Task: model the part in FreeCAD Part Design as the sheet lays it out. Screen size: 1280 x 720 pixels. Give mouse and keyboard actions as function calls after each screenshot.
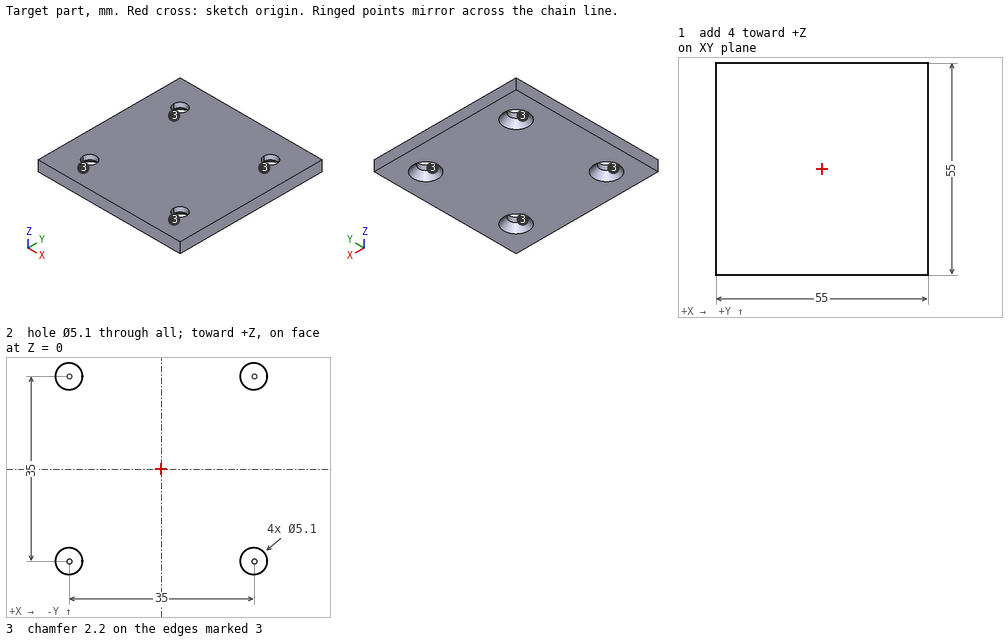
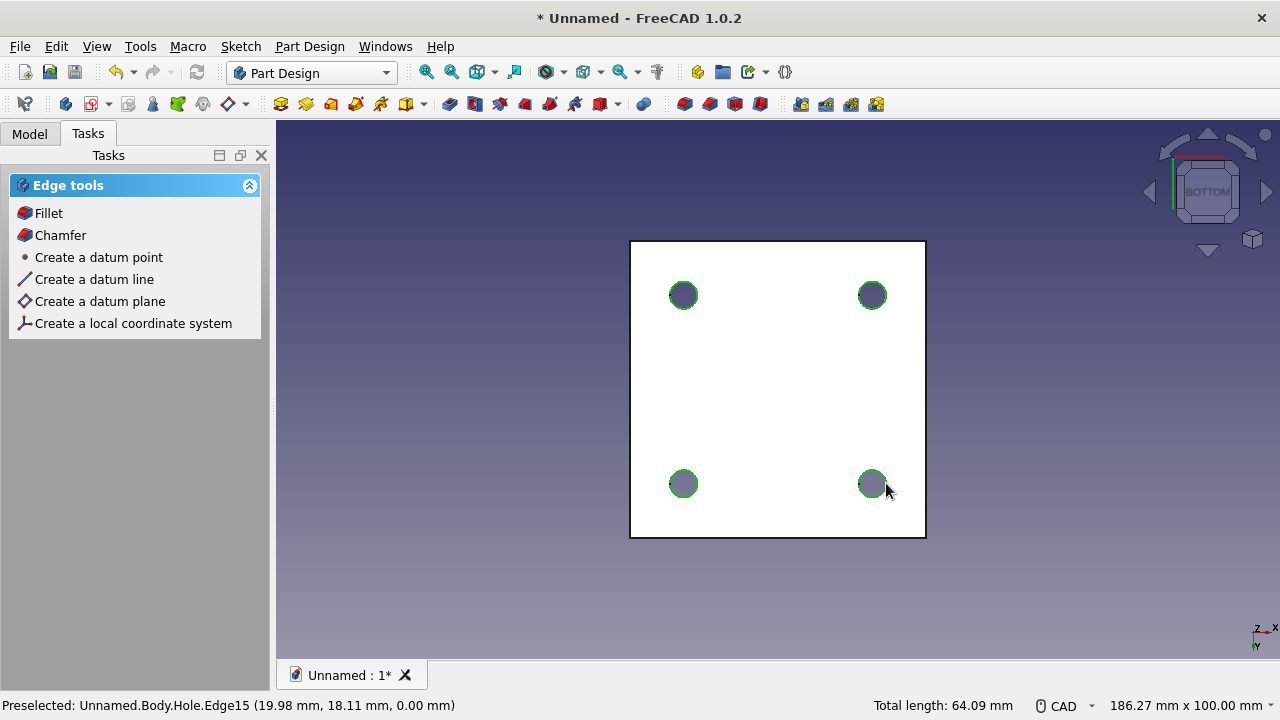
click(710, 104)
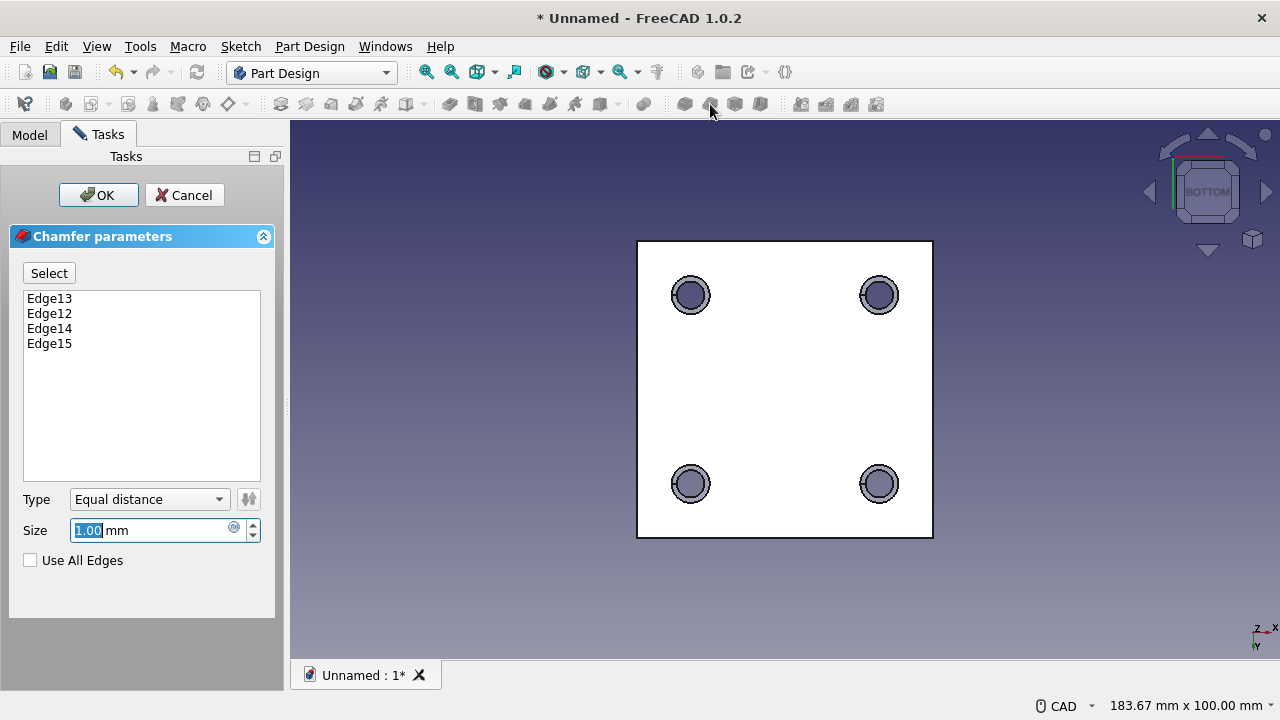
text(2.2)
key(Tab)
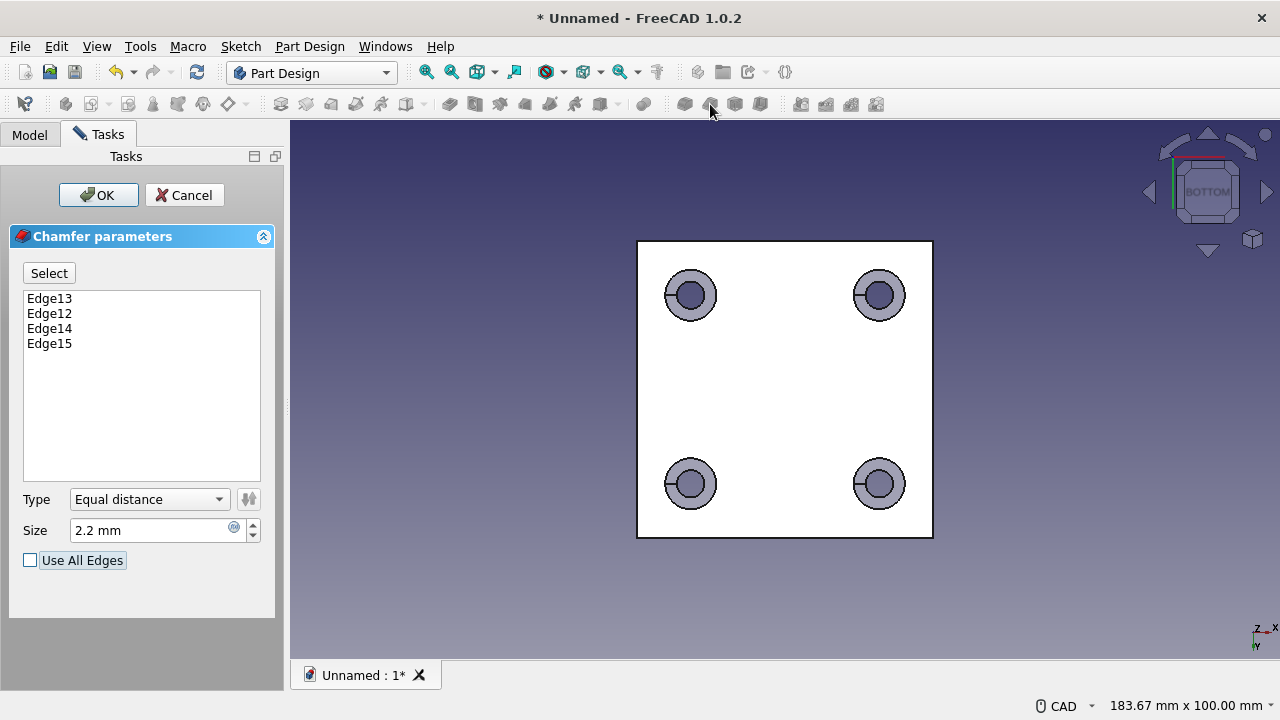
click(99, 195)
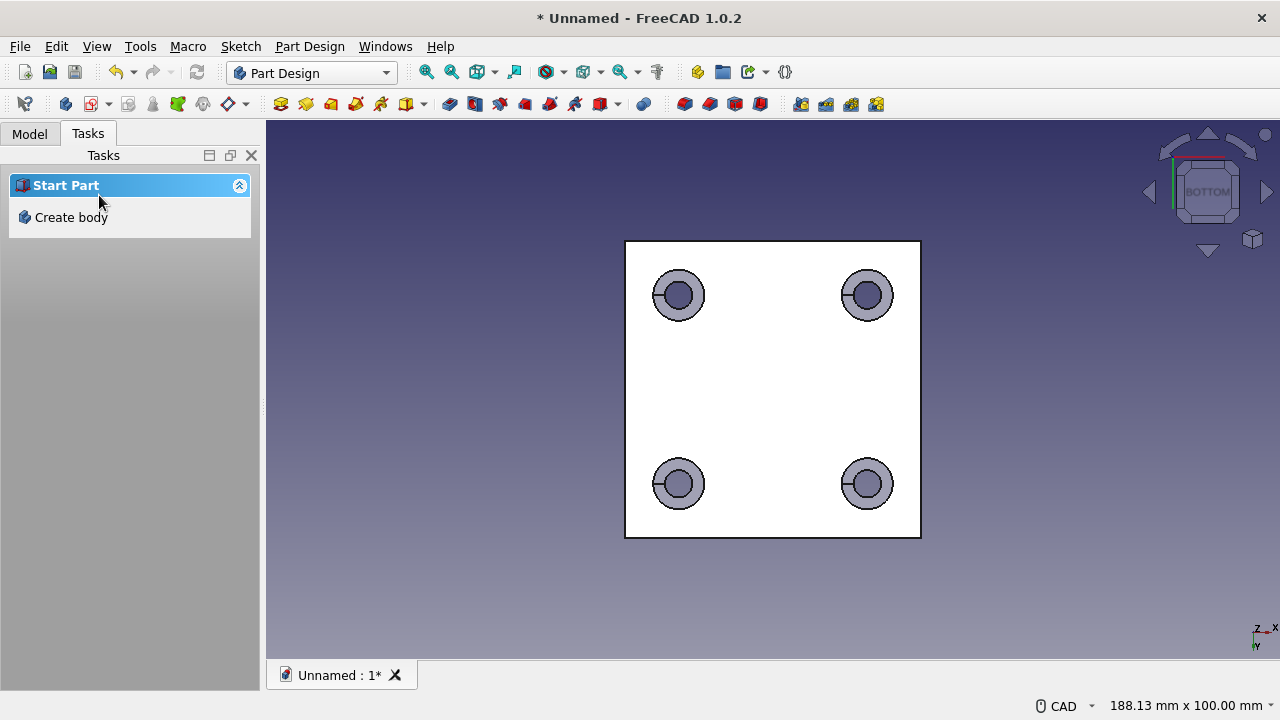
key(0)